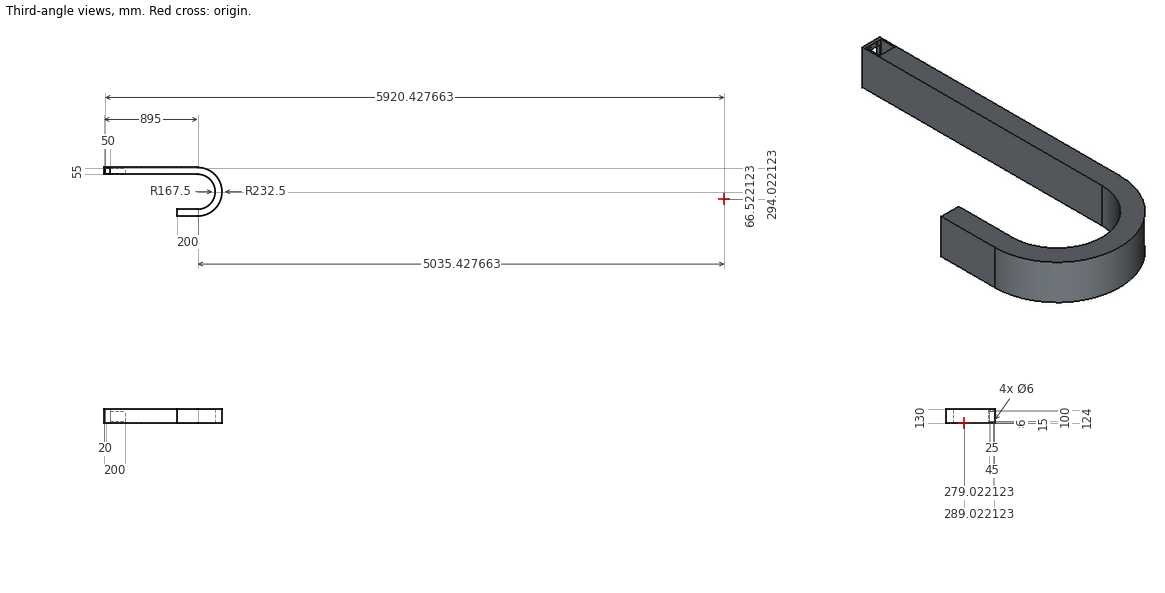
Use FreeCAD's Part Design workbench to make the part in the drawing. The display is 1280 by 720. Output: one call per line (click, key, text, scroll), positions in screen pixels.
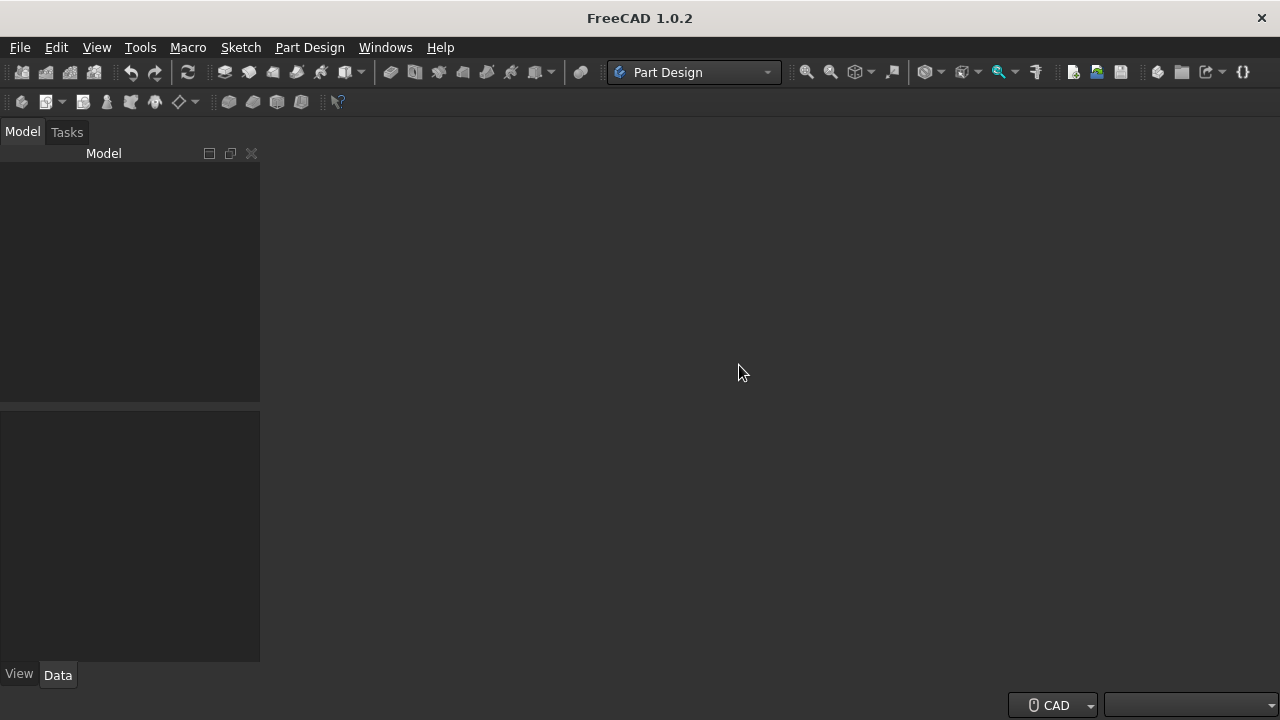
key(ctrl+n)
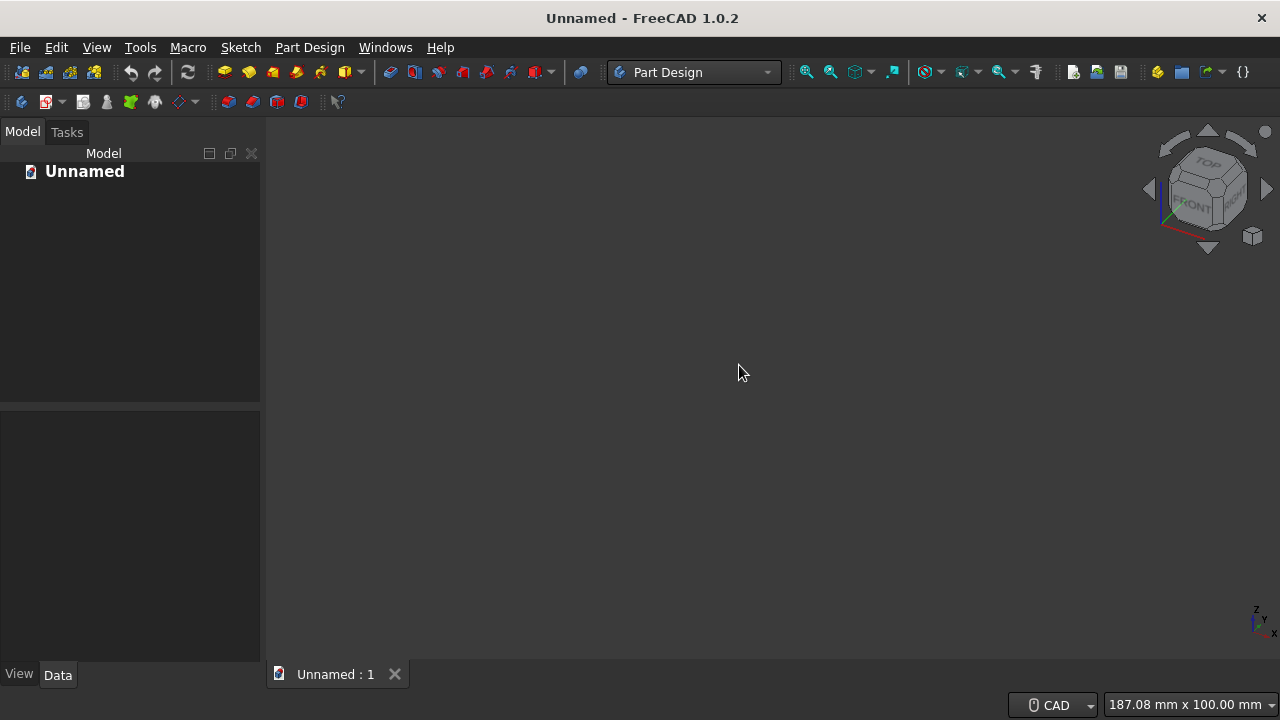
click(46, 102)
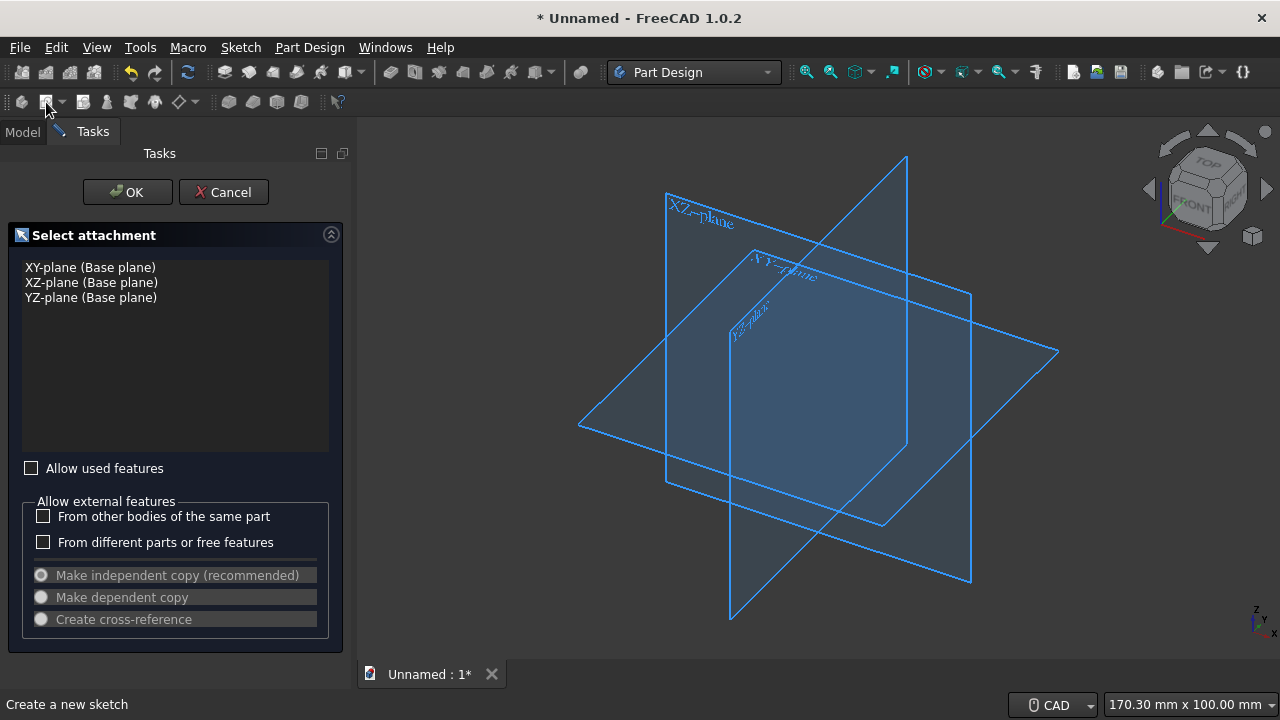
click(82, 268)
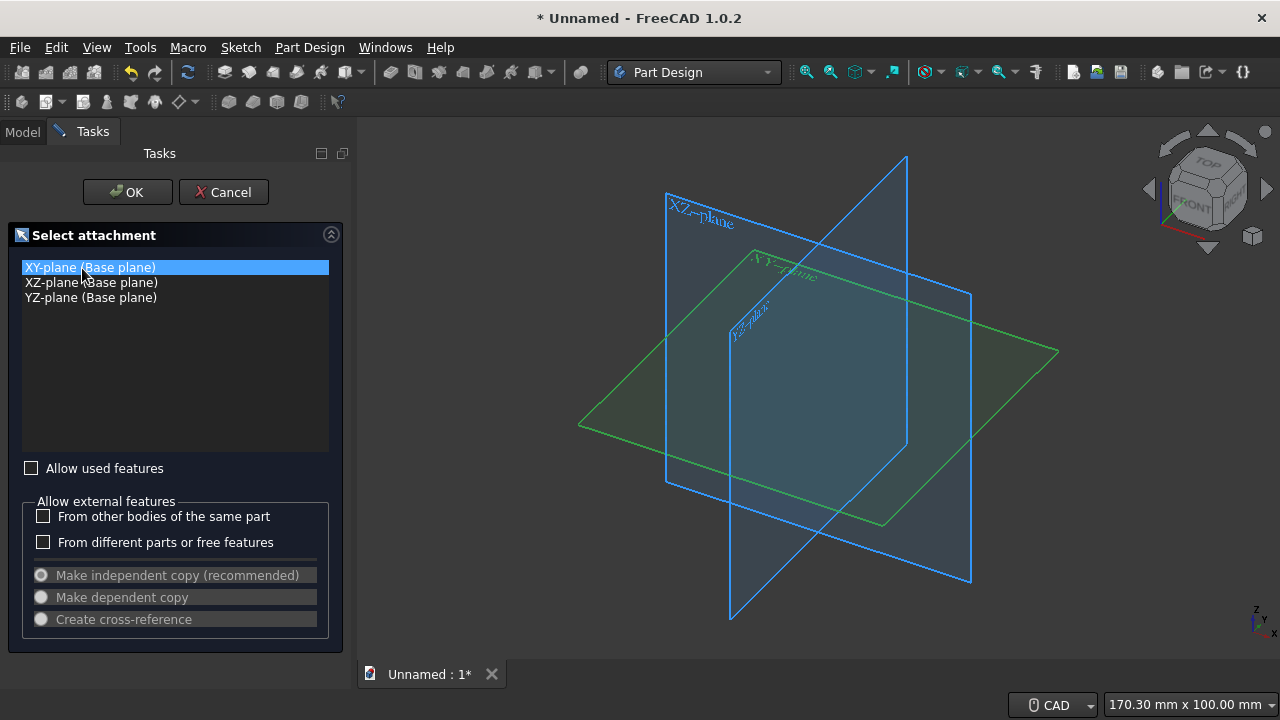
click(128, 192)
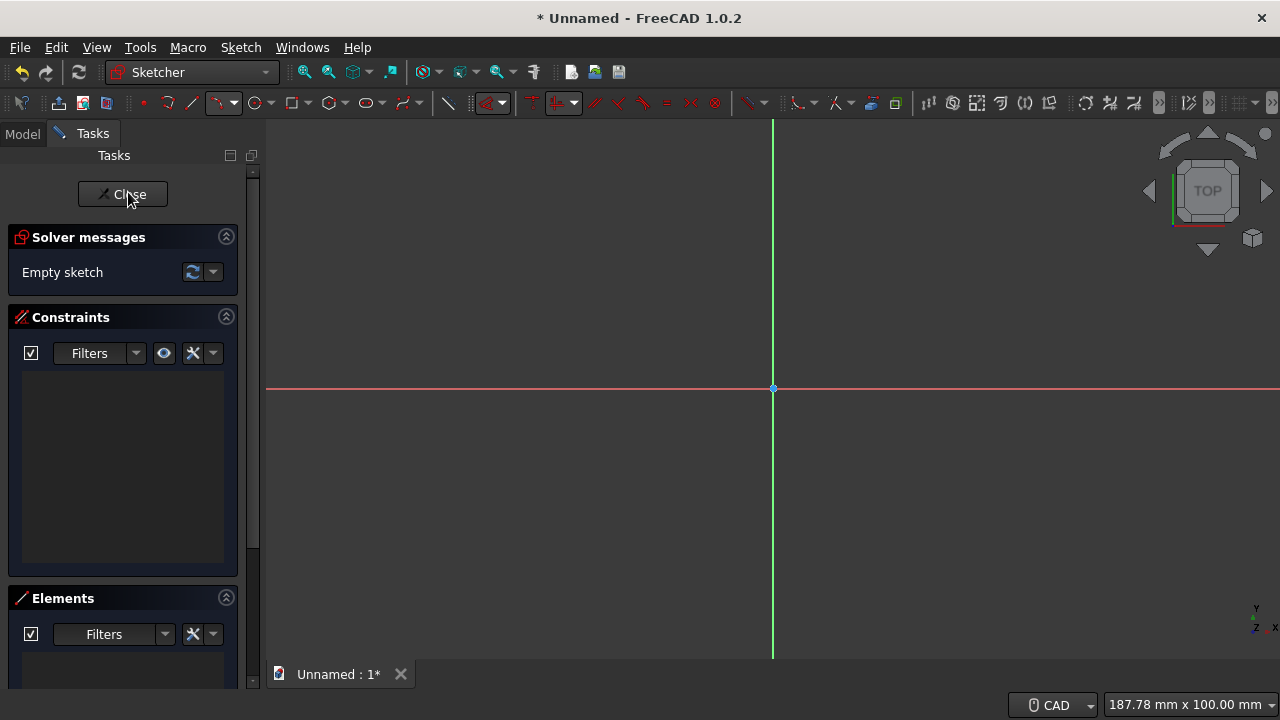
scroll(704, 389, down, 12)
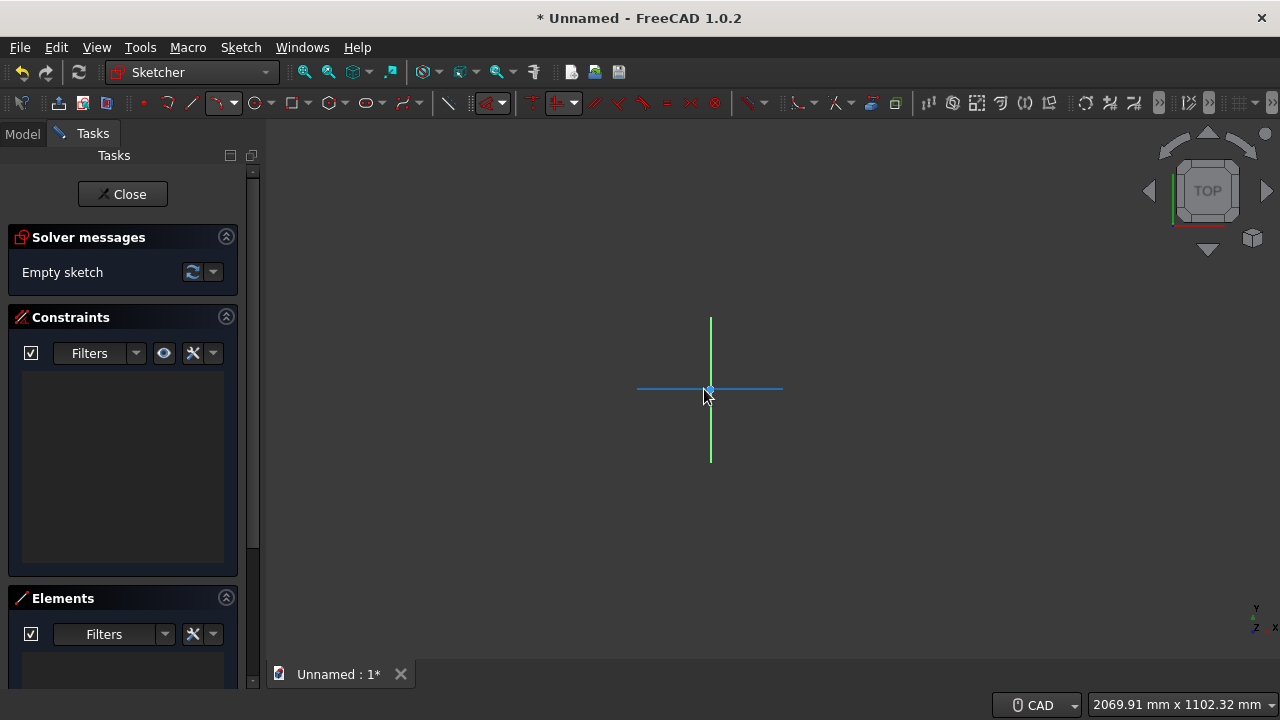
scroll(704, 389, down, 5)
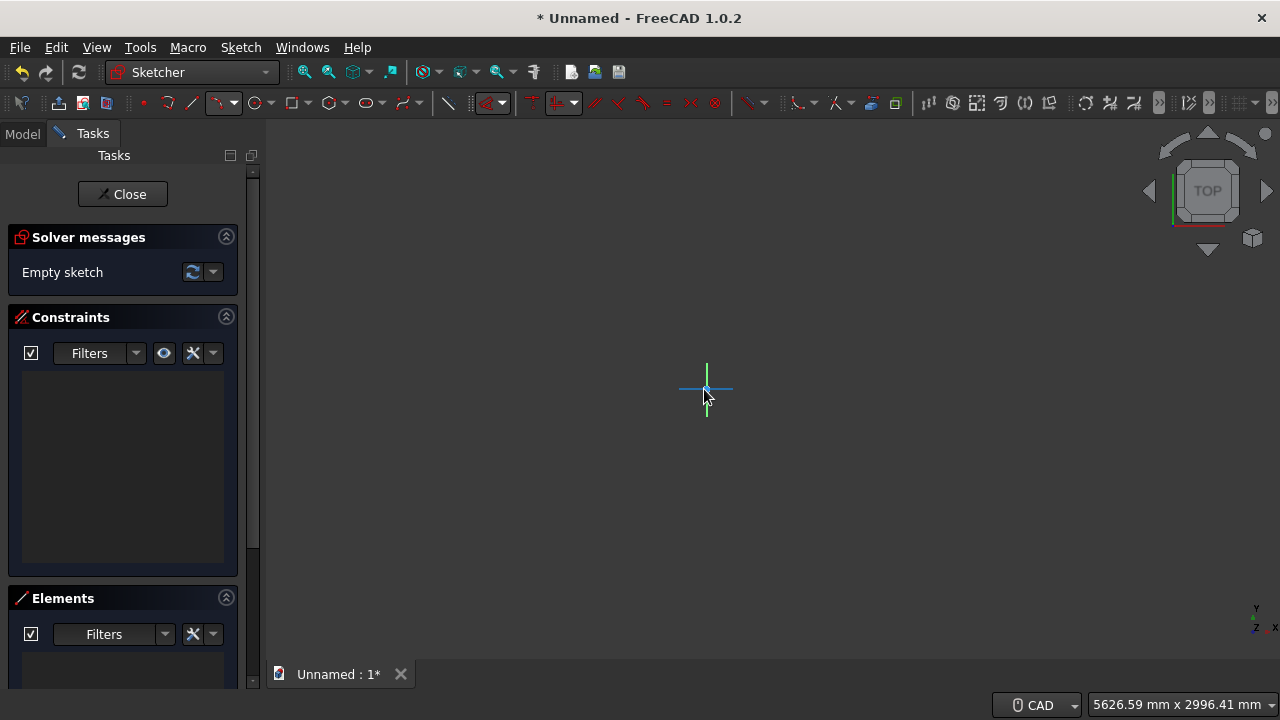
scroll(704, 389, down, 5)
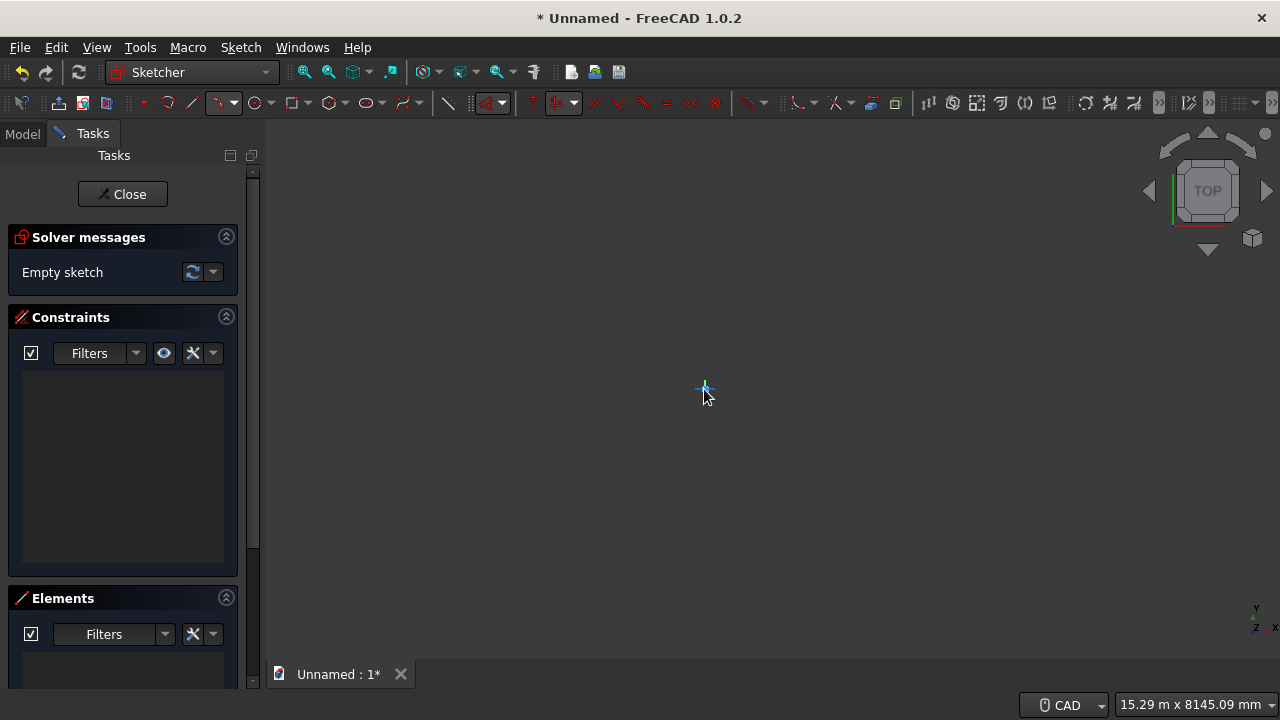
scroll(294, 384, up, 10)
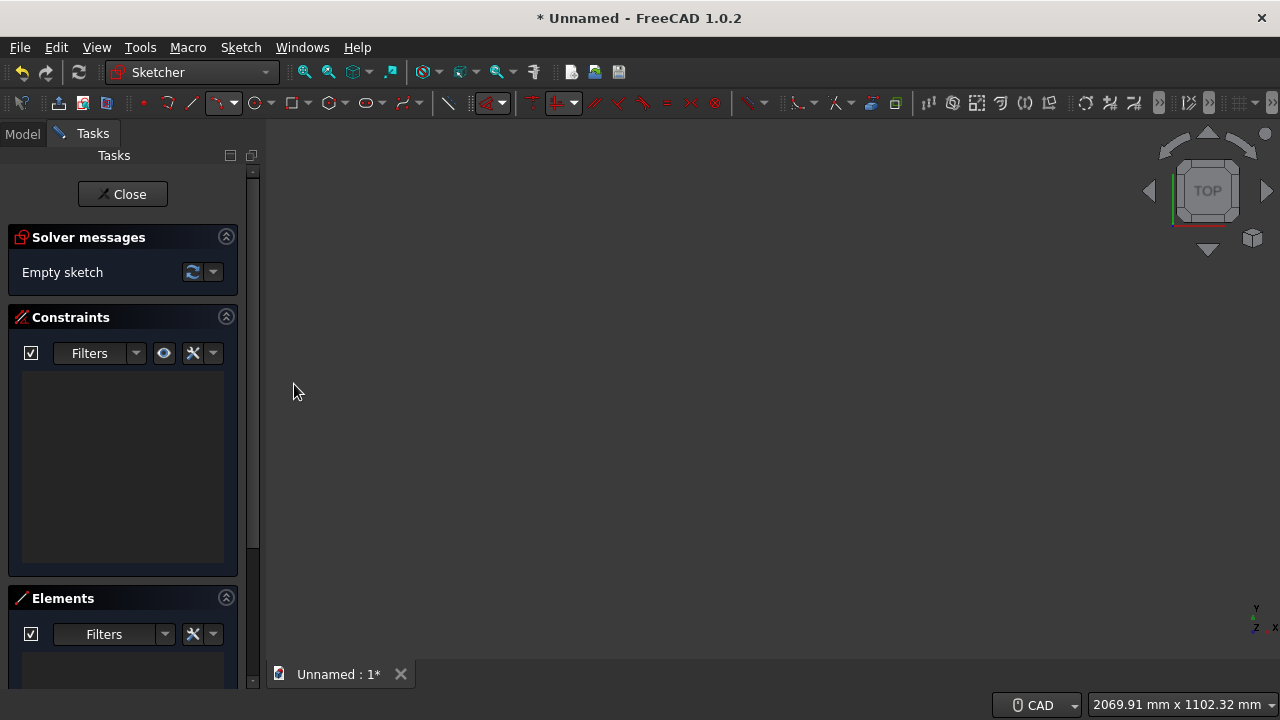
click(168, 104)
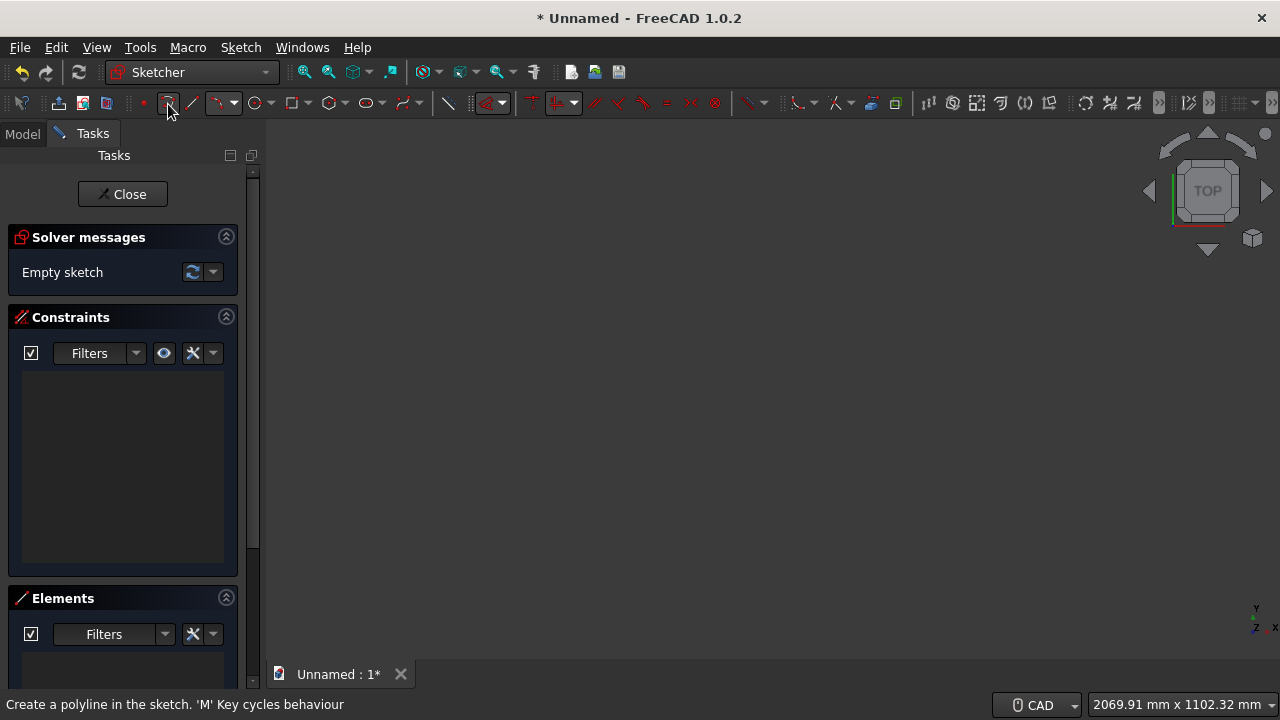
click(866, 471)
click(768, 471)
click(768, 503)
click(866, 503)
right_click(866, 503)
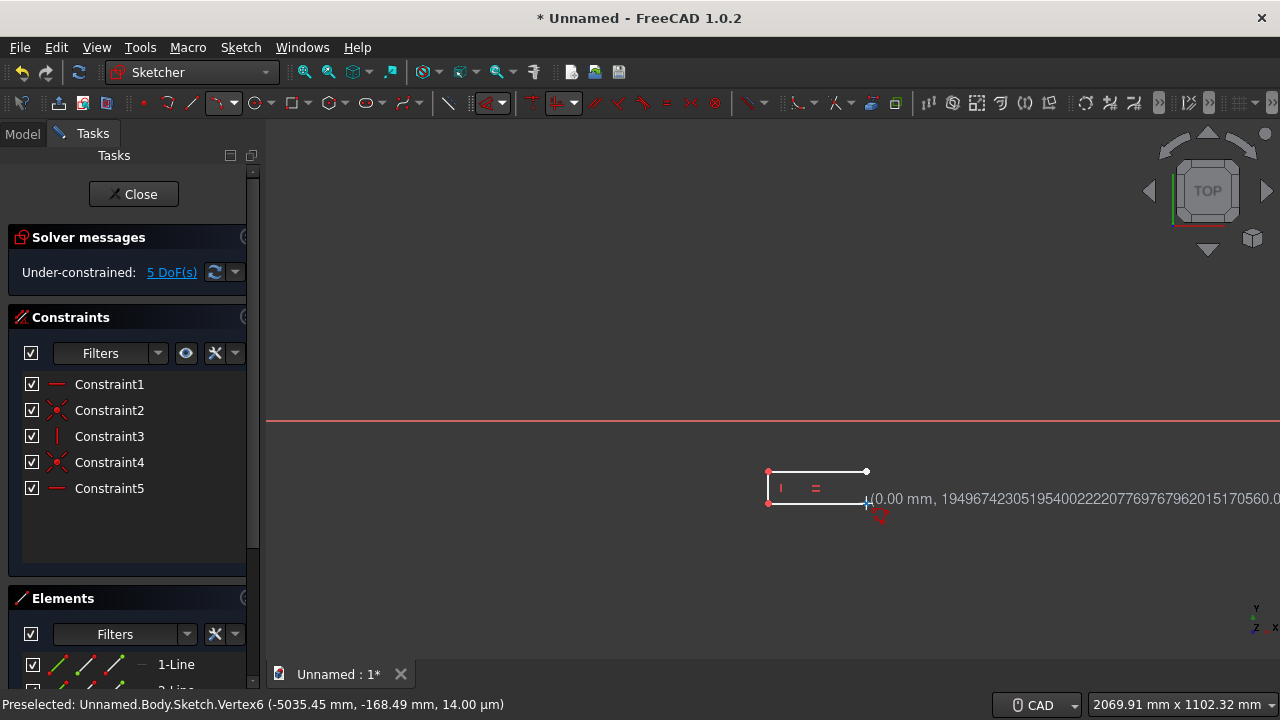
click(866, 275)
click(428, 275)
click(428, 307)
click(866, 307)
right_click(866, 307)